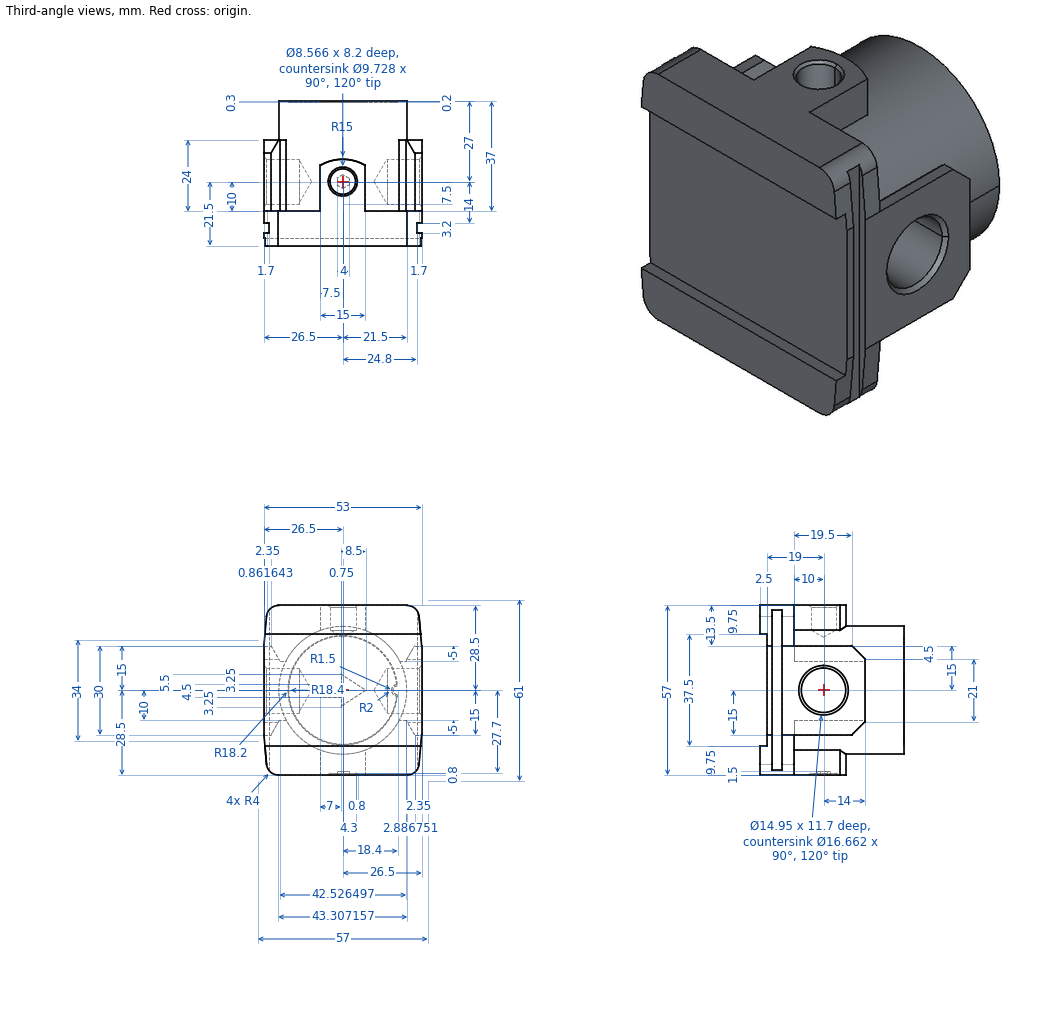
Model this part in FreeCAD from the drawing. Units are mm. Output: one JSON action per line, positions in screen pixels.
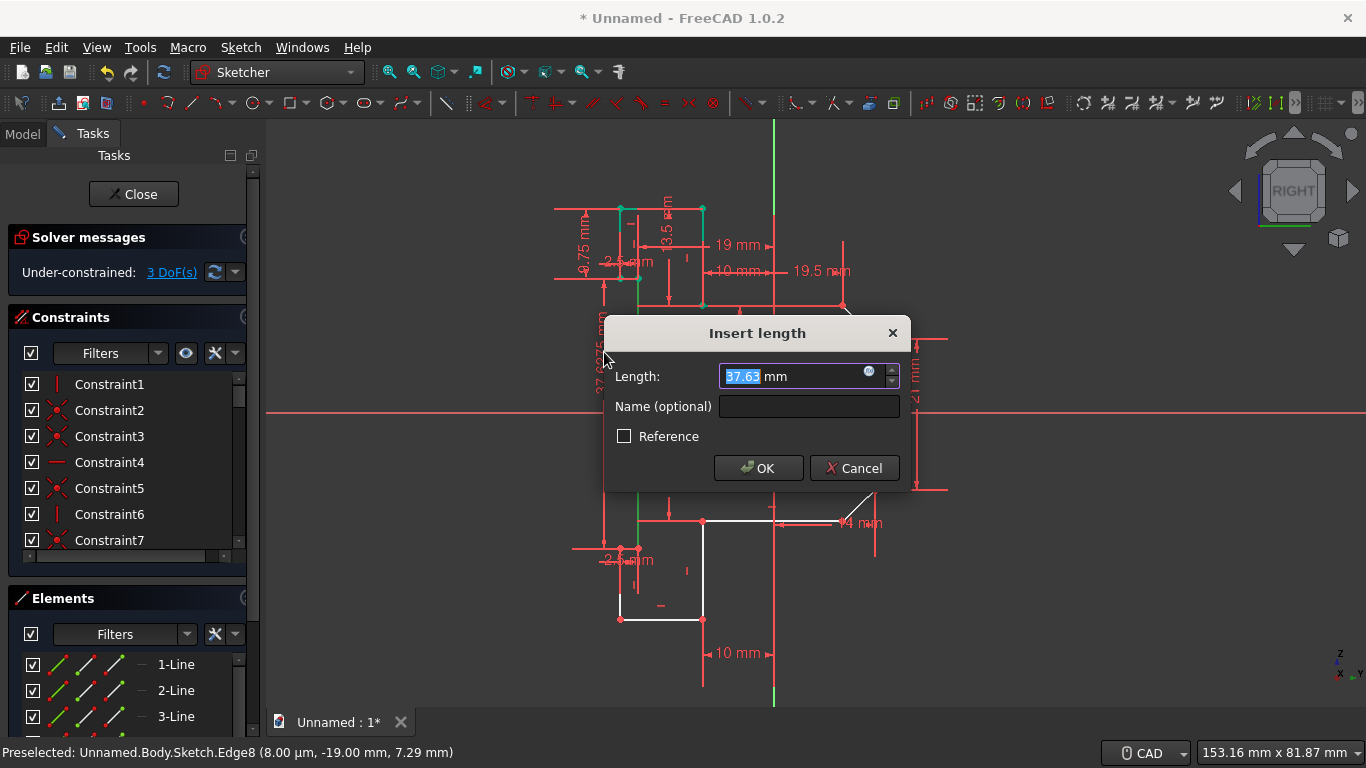
{"action": "type", "text": "37.5"}
{"action": "key", "text": "Return"}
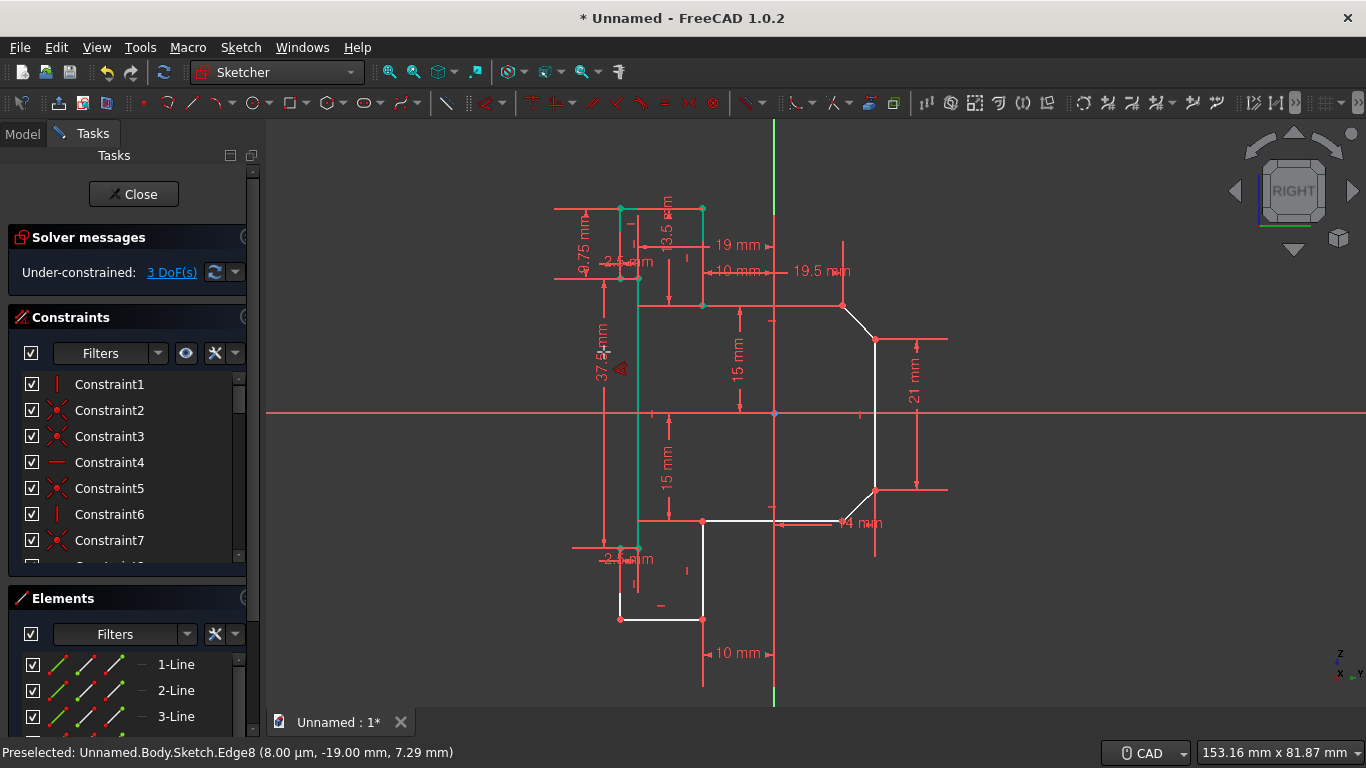
{"action": "left_click", "coordinate": [620, 570]}
{"action": "left_click", "coordinate": [586, 584]}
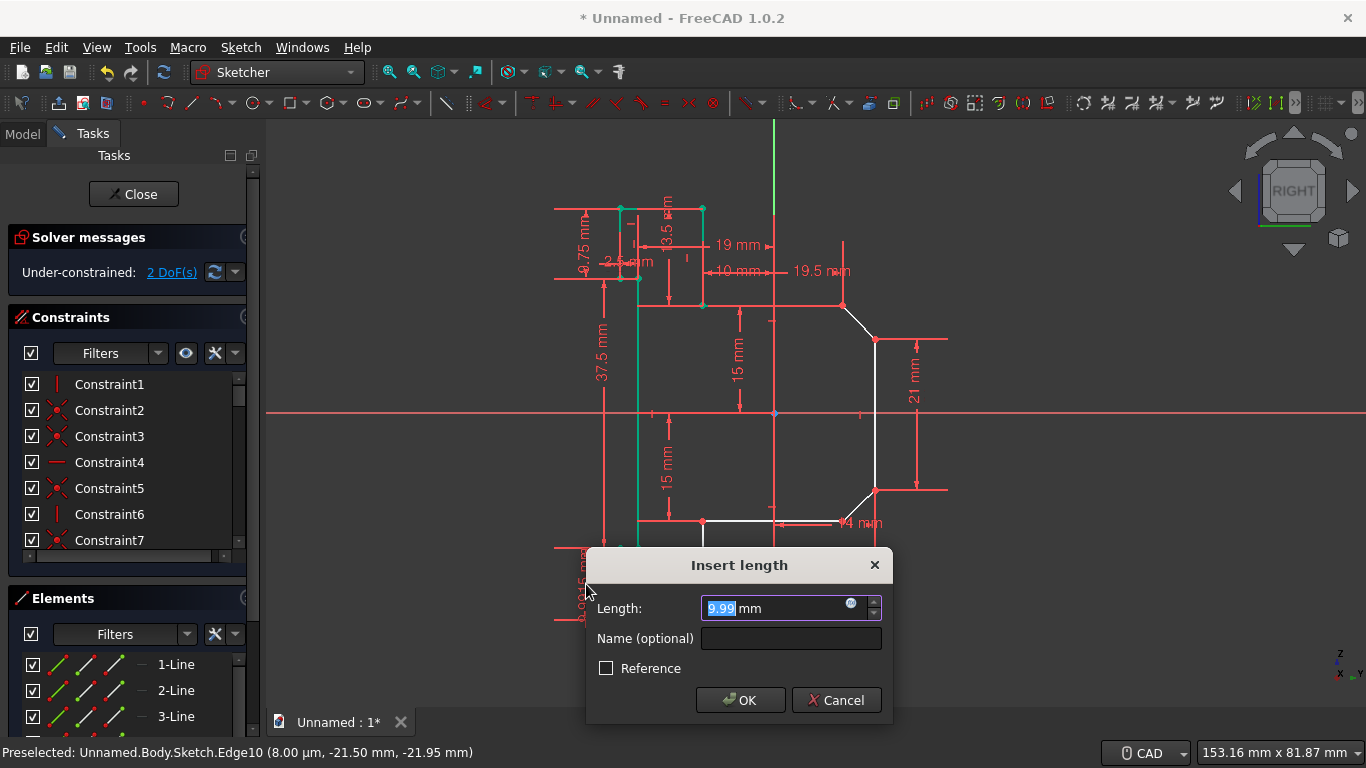
{"action": "type", "text": "9.75"}
{"action": "key", "text": "Return"}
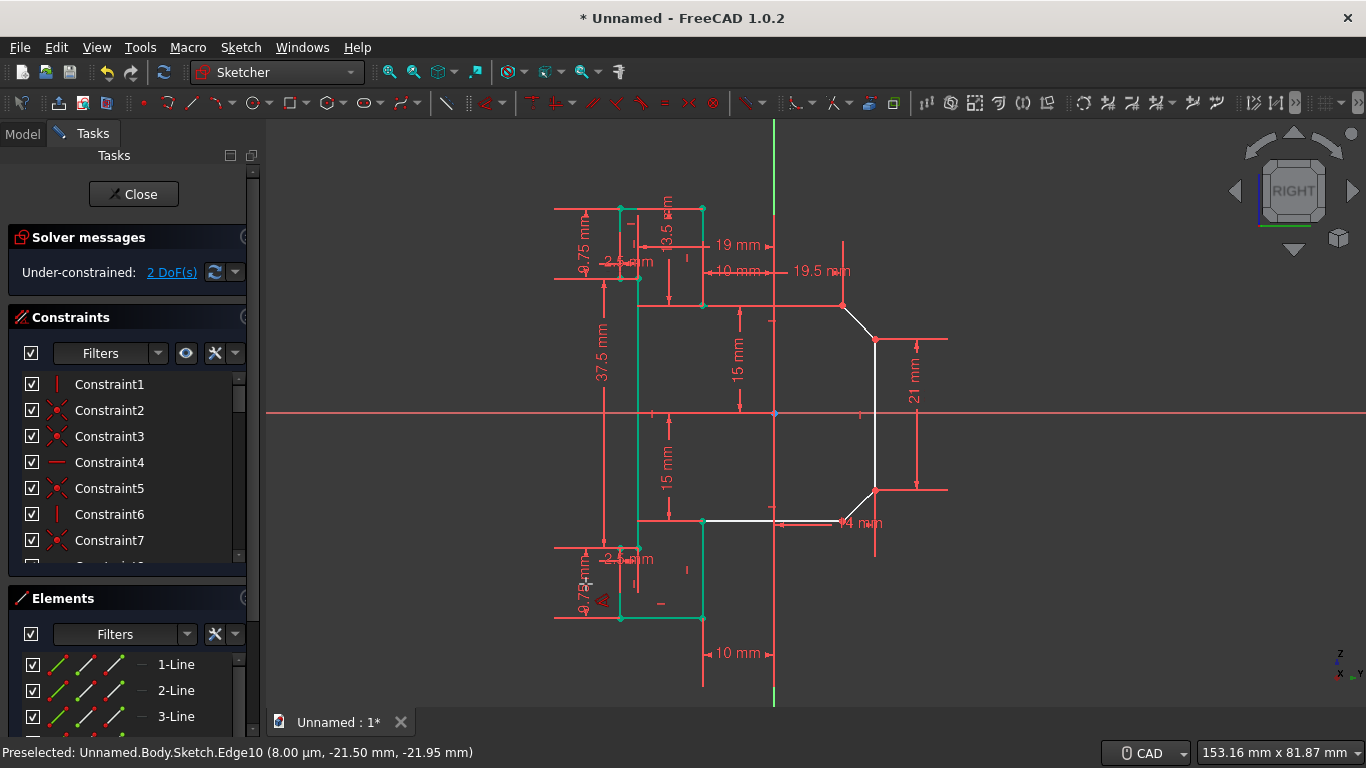
{"action": "left_click", "coordinate": [745, 521]}
{"action": "left_click", "coordinate": [741, 555]}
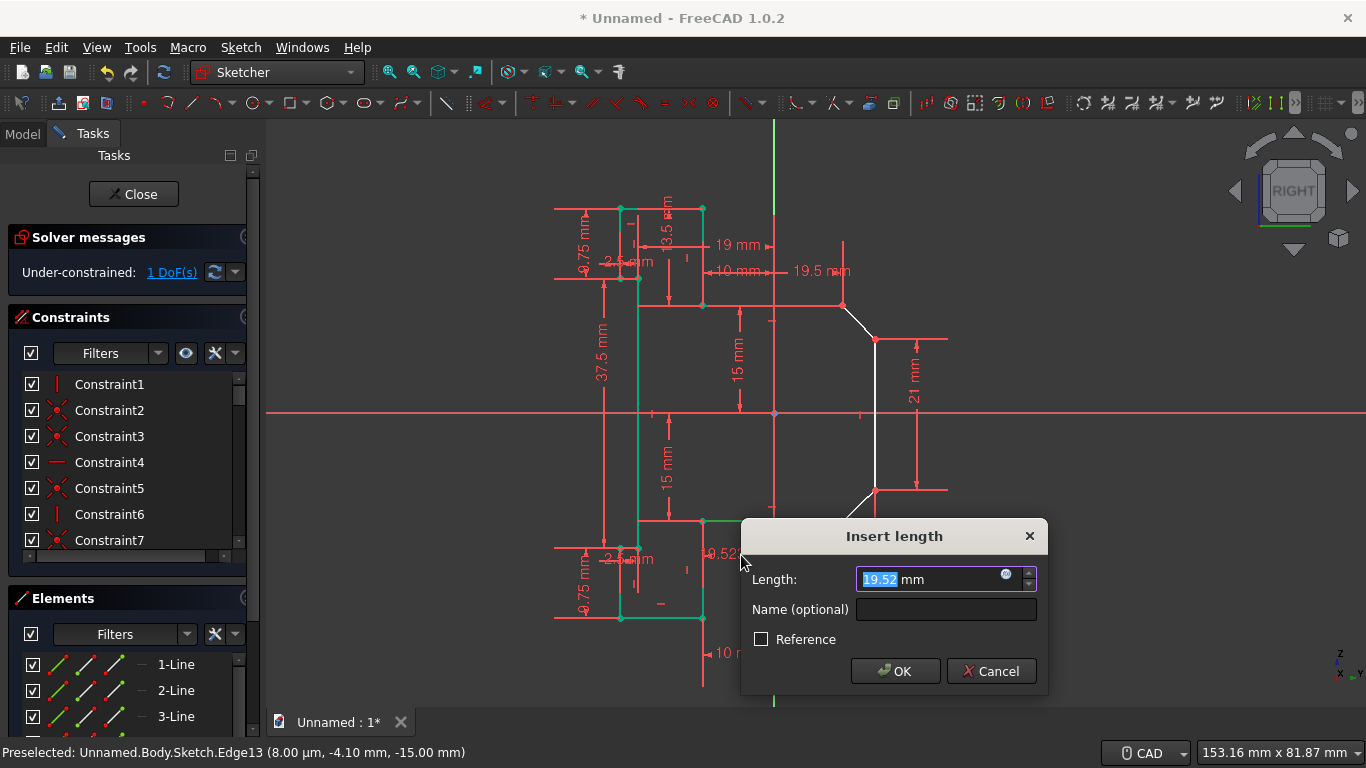
{"action": "type", "text": "19.5"}
{"action": "key", "text": "Return"}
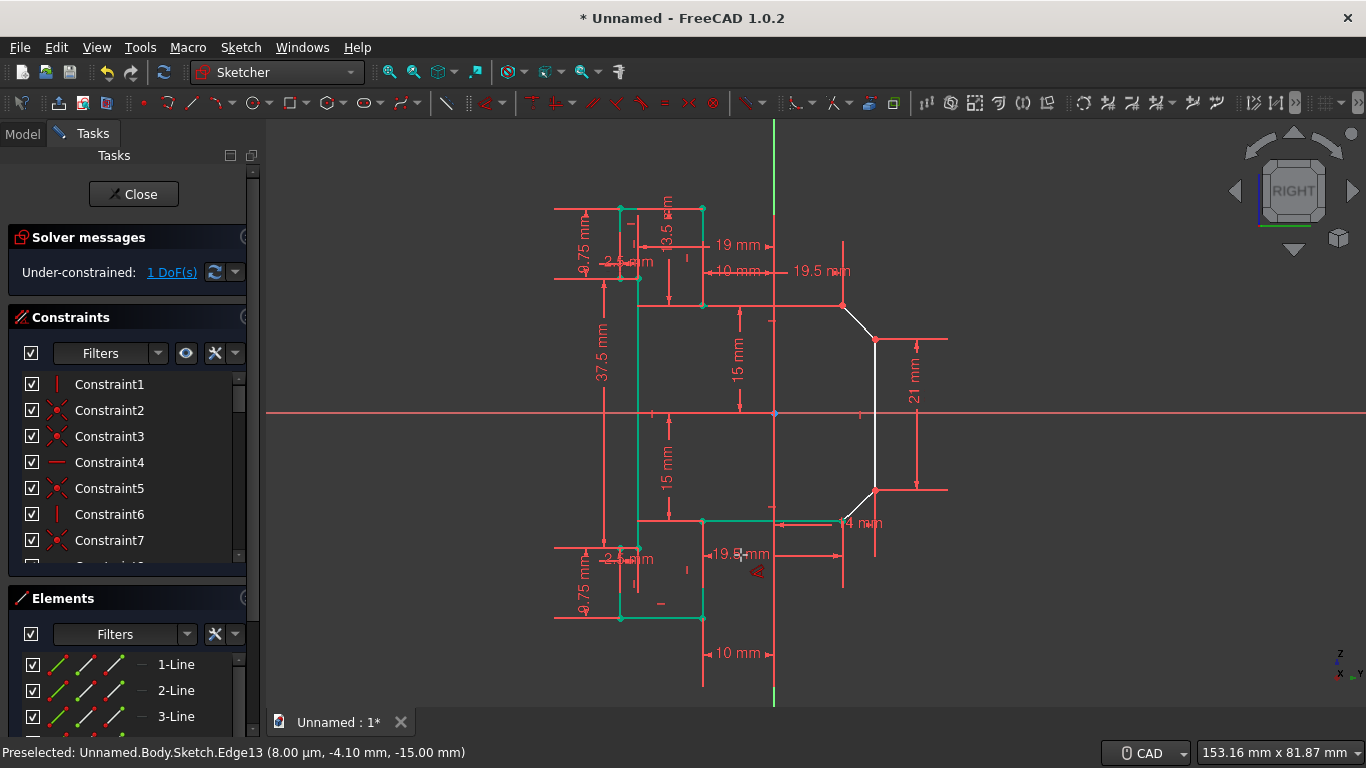
{"action": "scroll", "coordinate": [865, 329], "scroll_direction": "up", "scroll_amount": 2}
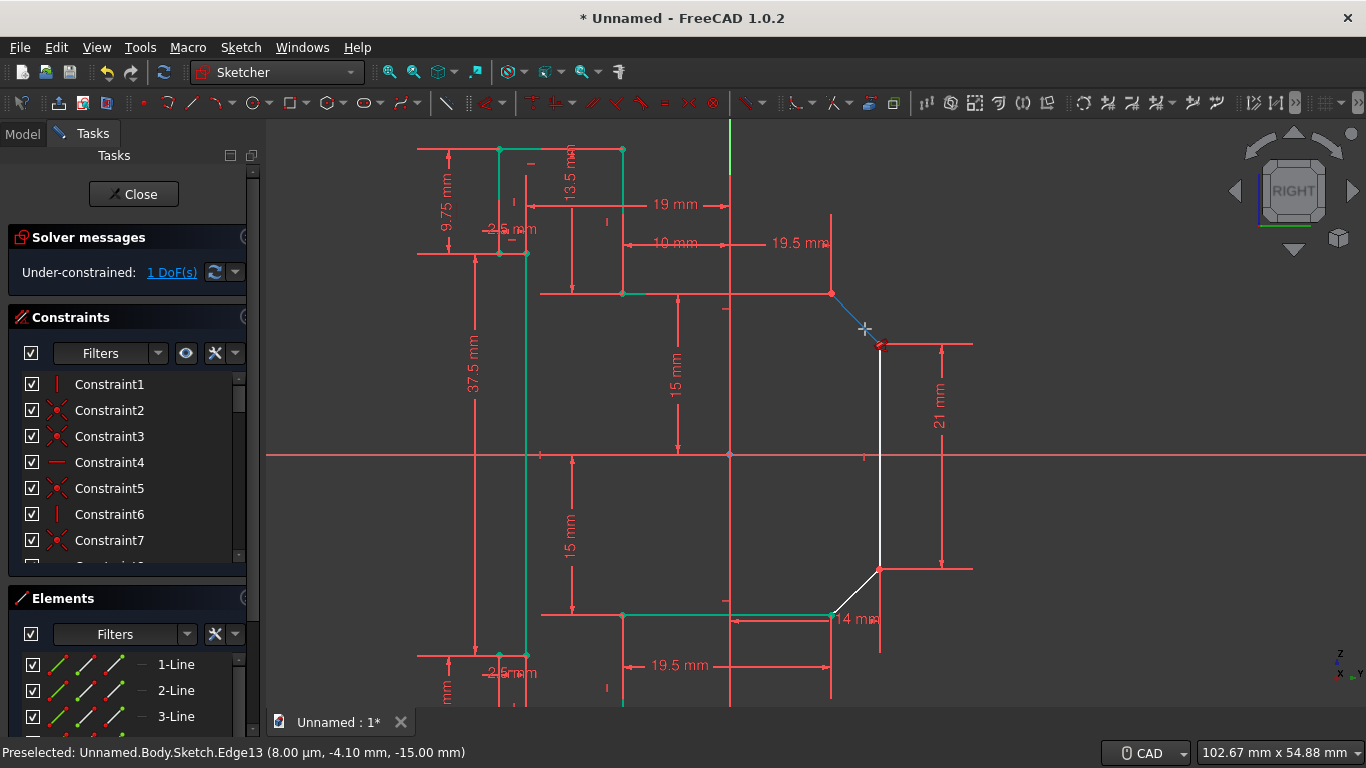
{"action": "left_click", "coordinate": [865, 329]}
{"action": "left_click", "coordinate": [914, 319]}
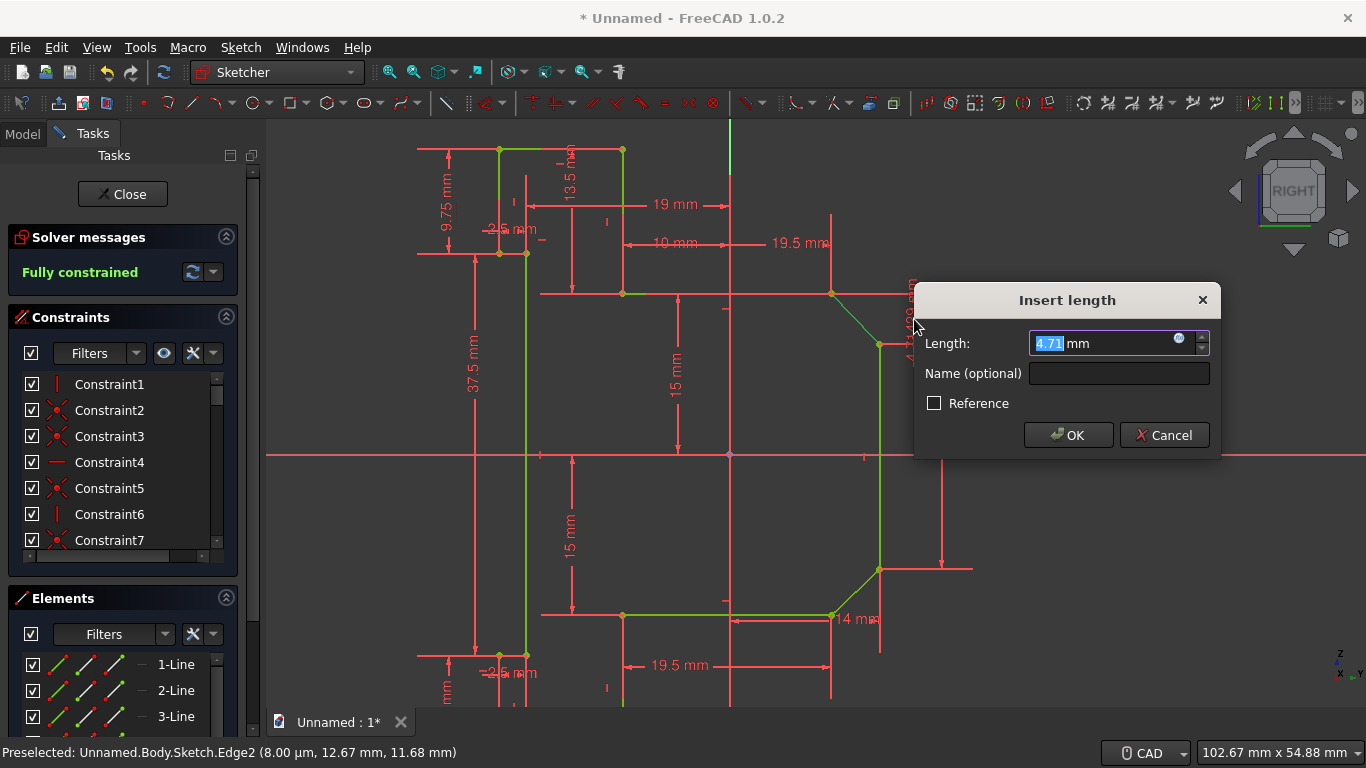
{"action": "type", "text": "4.5"}
{"action": "key", "text": "Return"}
{"action": "key", "text": "Escape"}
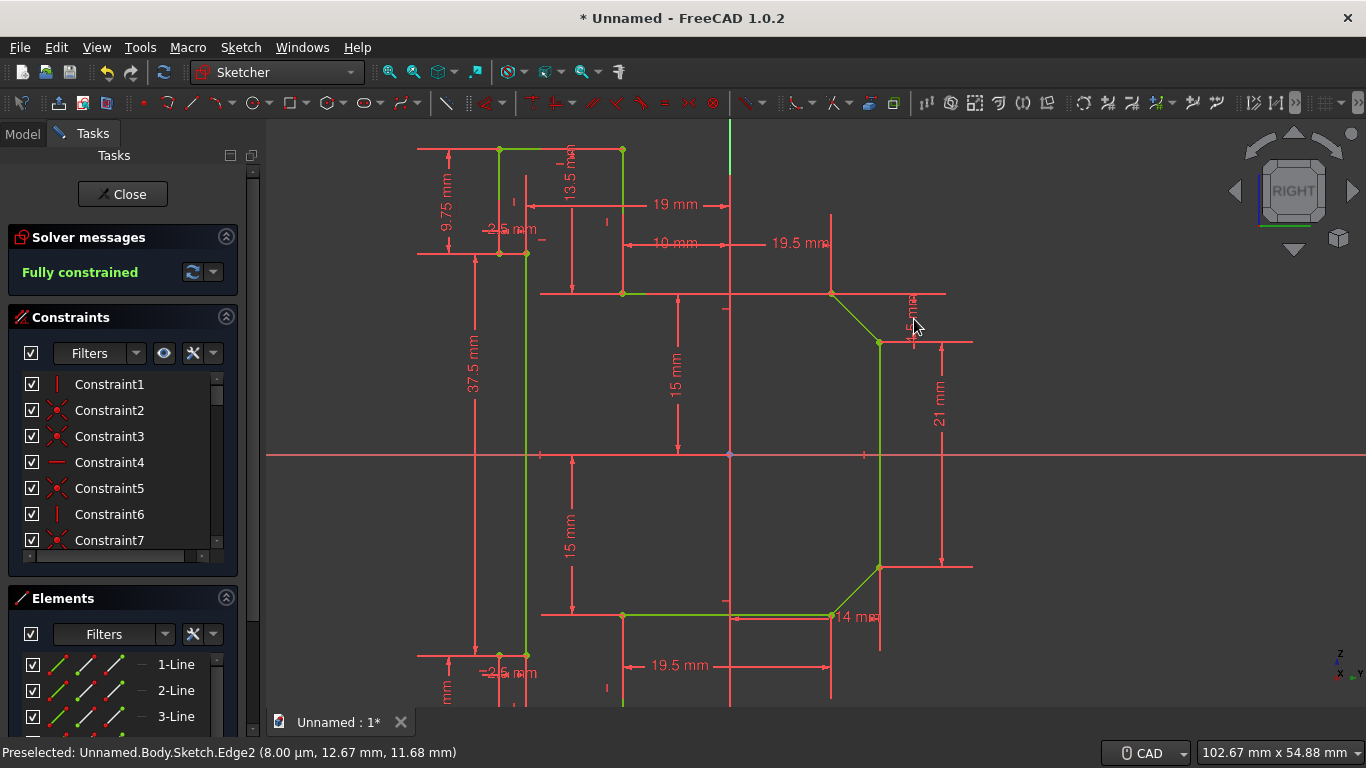
{"action": "left_click", "coordinate": [123, 194]}